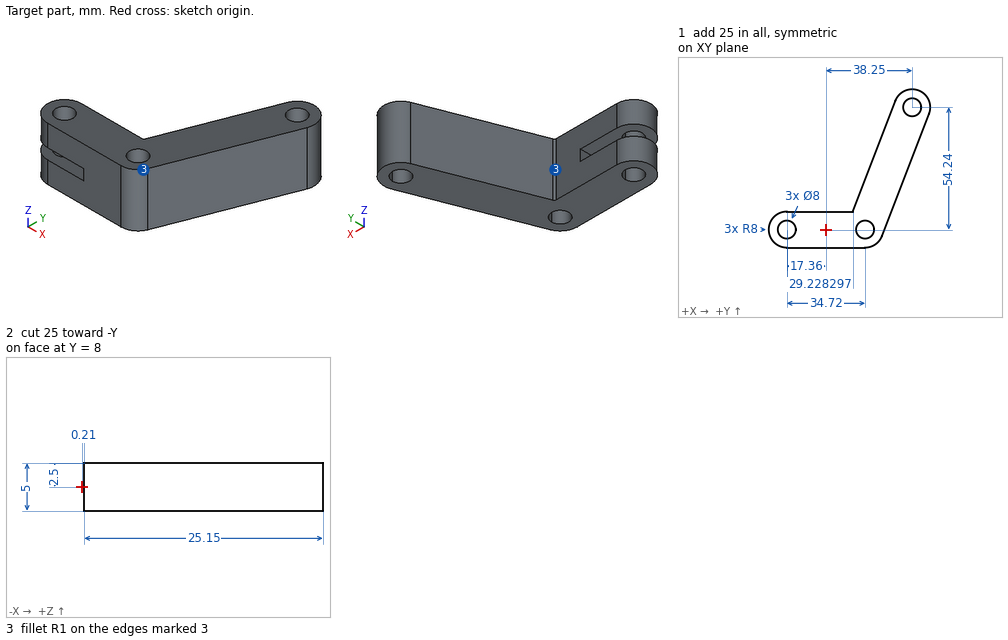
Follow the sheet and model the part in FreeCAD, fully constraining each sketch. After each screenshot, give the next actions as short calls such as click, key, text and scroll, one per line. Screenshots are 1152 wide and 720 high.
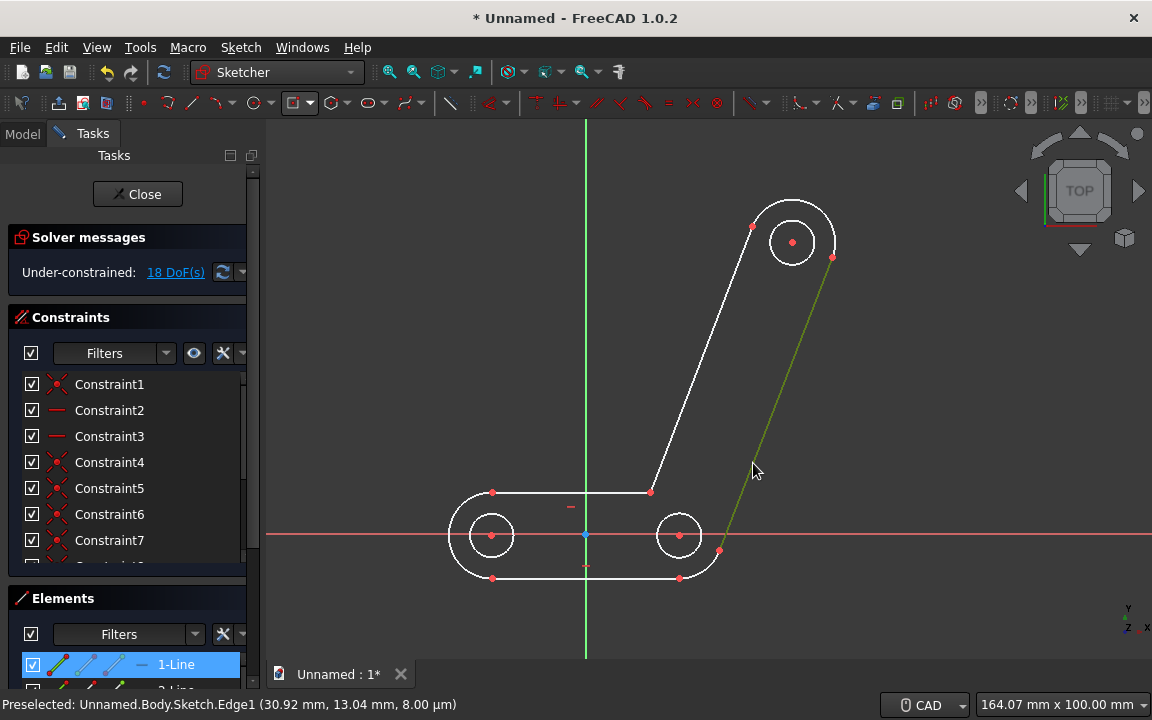
click(828, 219)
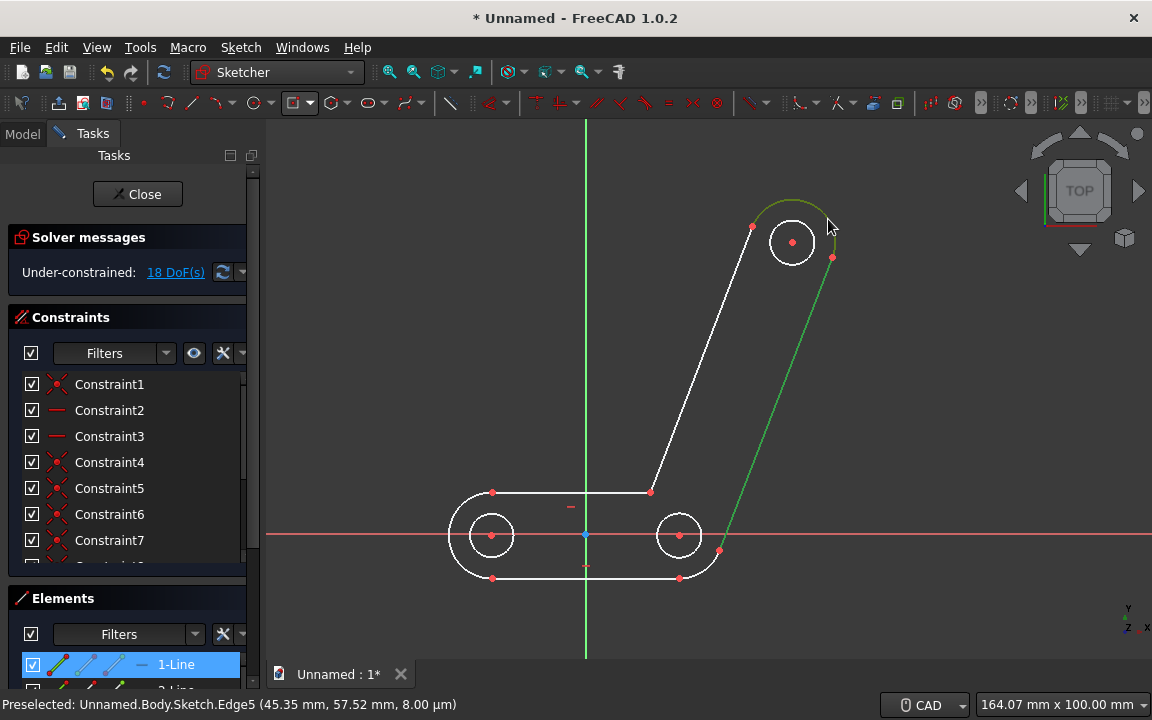
click(646, 104)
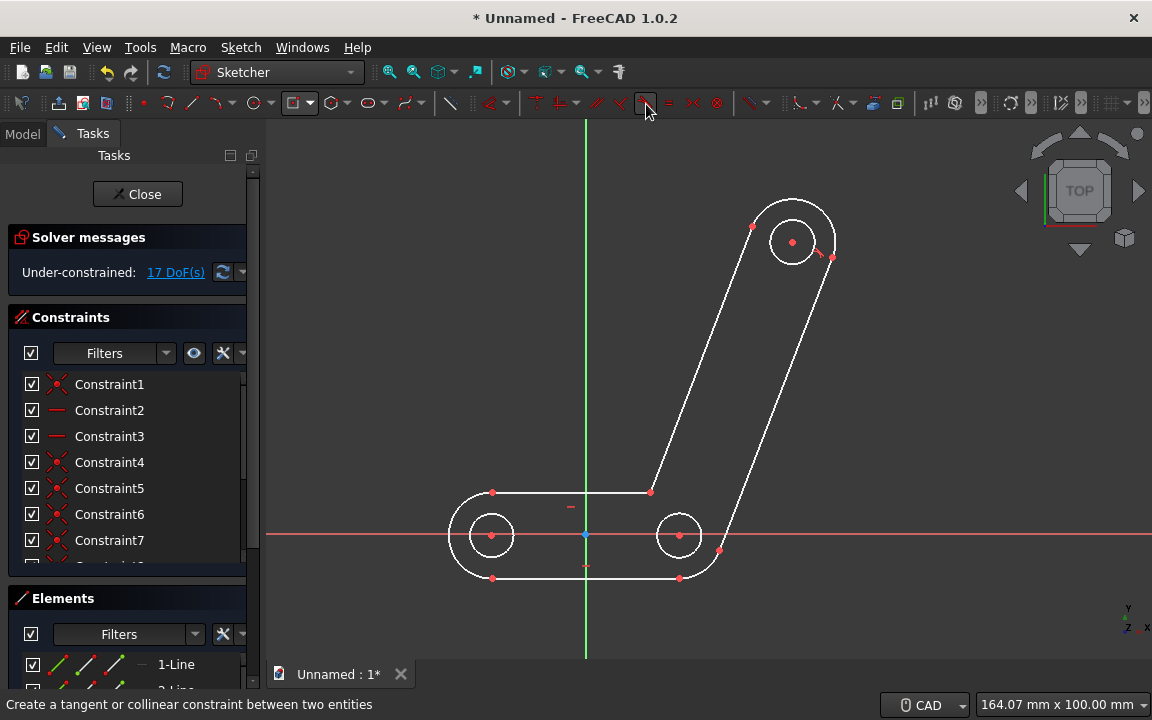
click(753, 463)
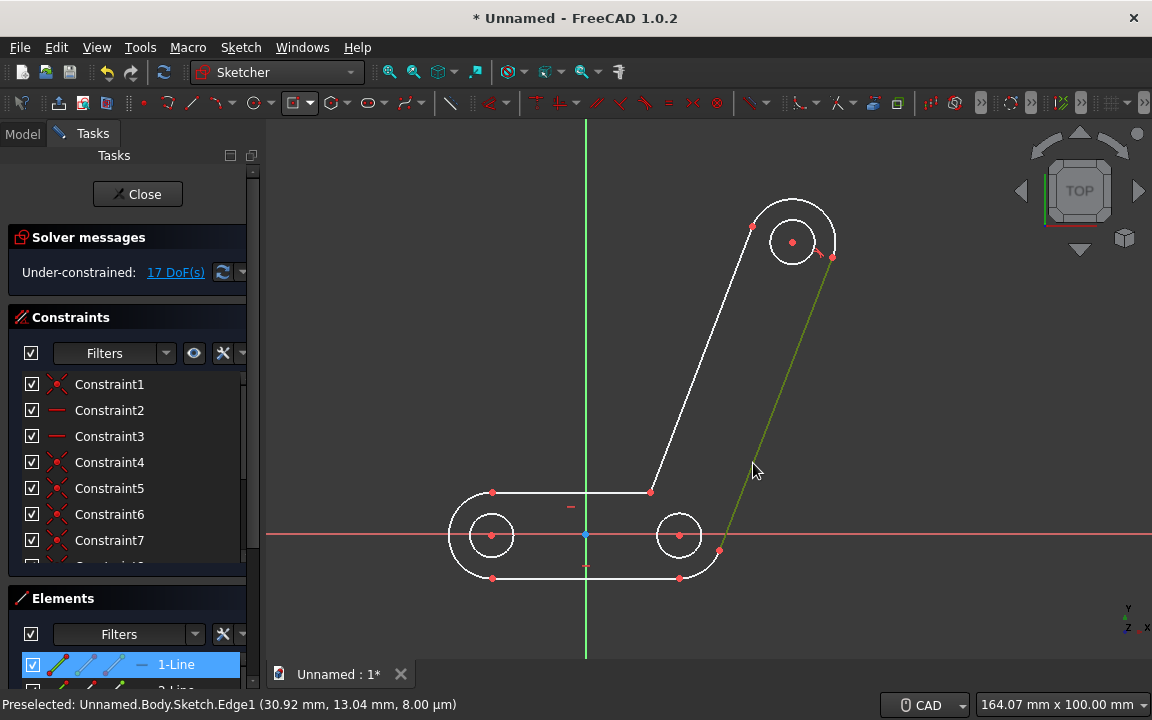
click(695, 576)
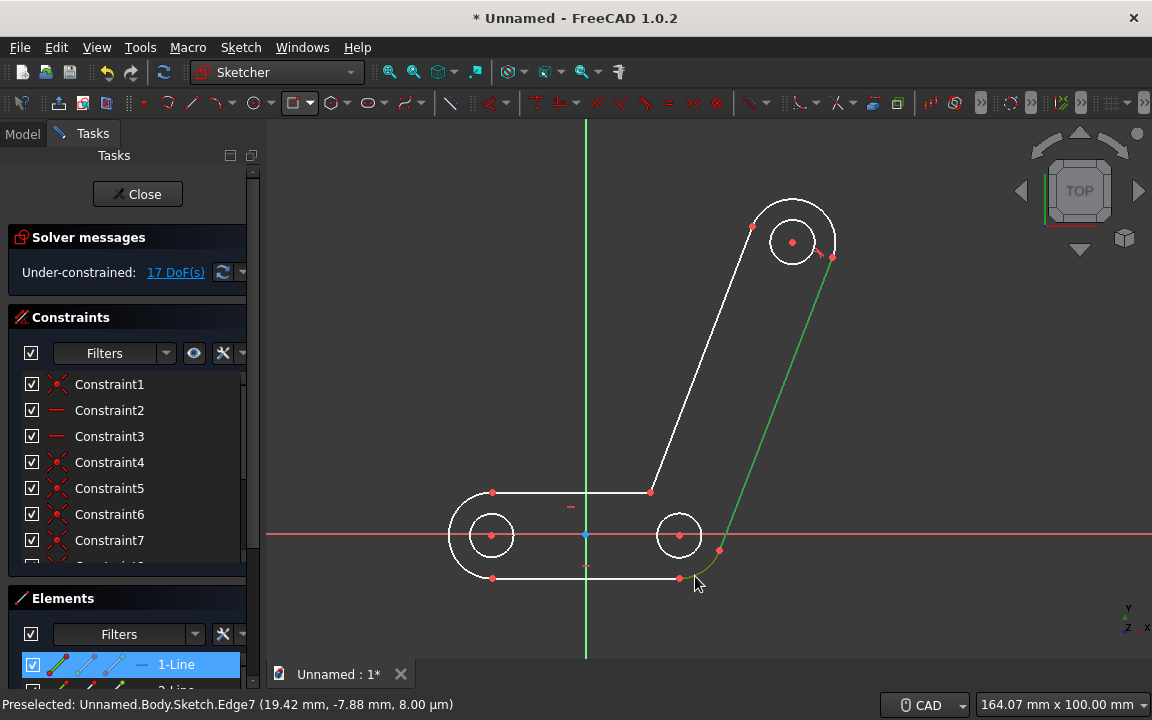
click(646, 104)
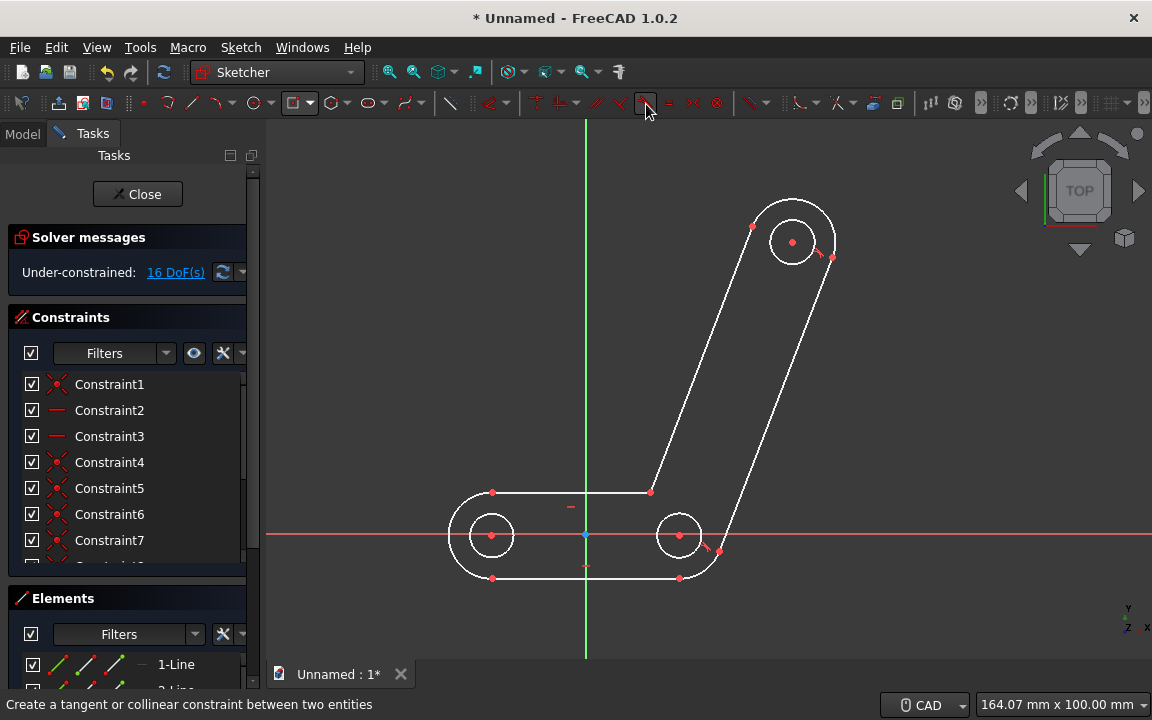
click(722, 306)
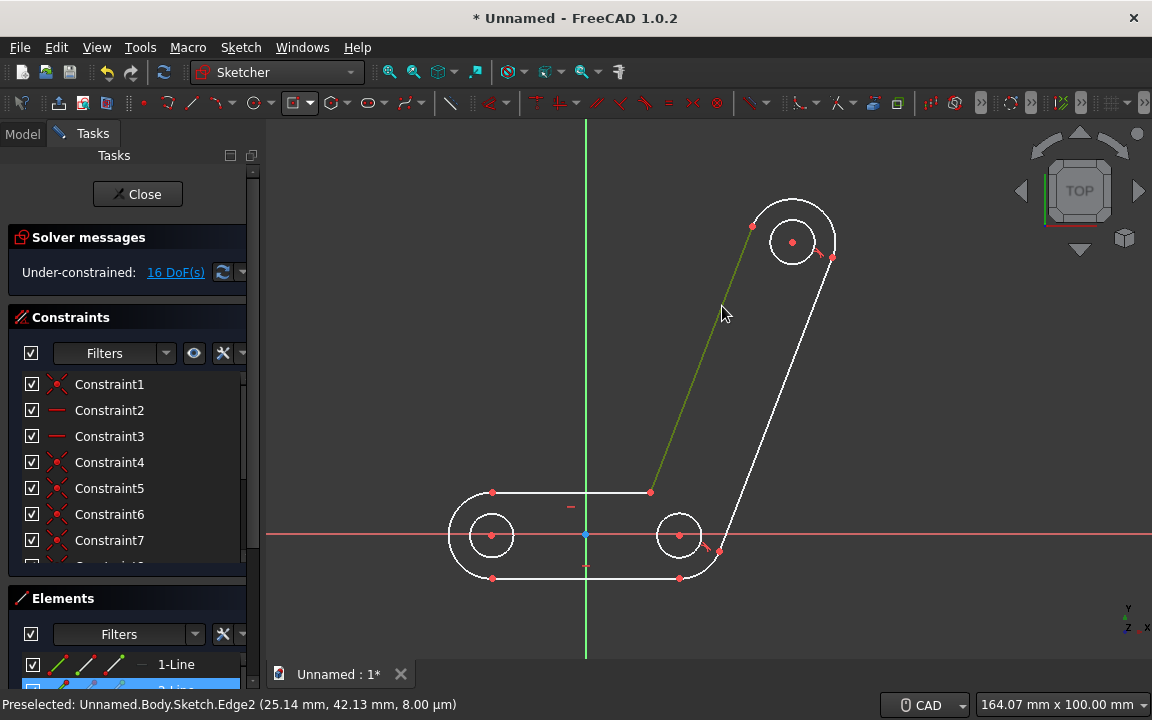
click(829, 219)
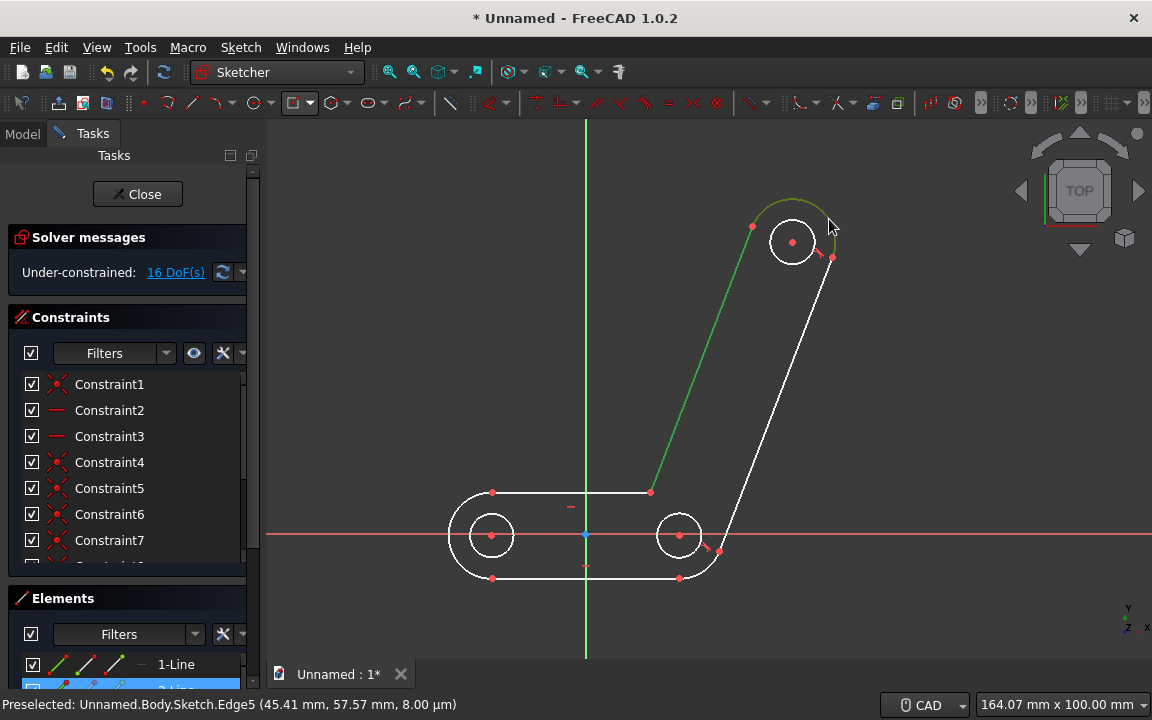
click(646, 104)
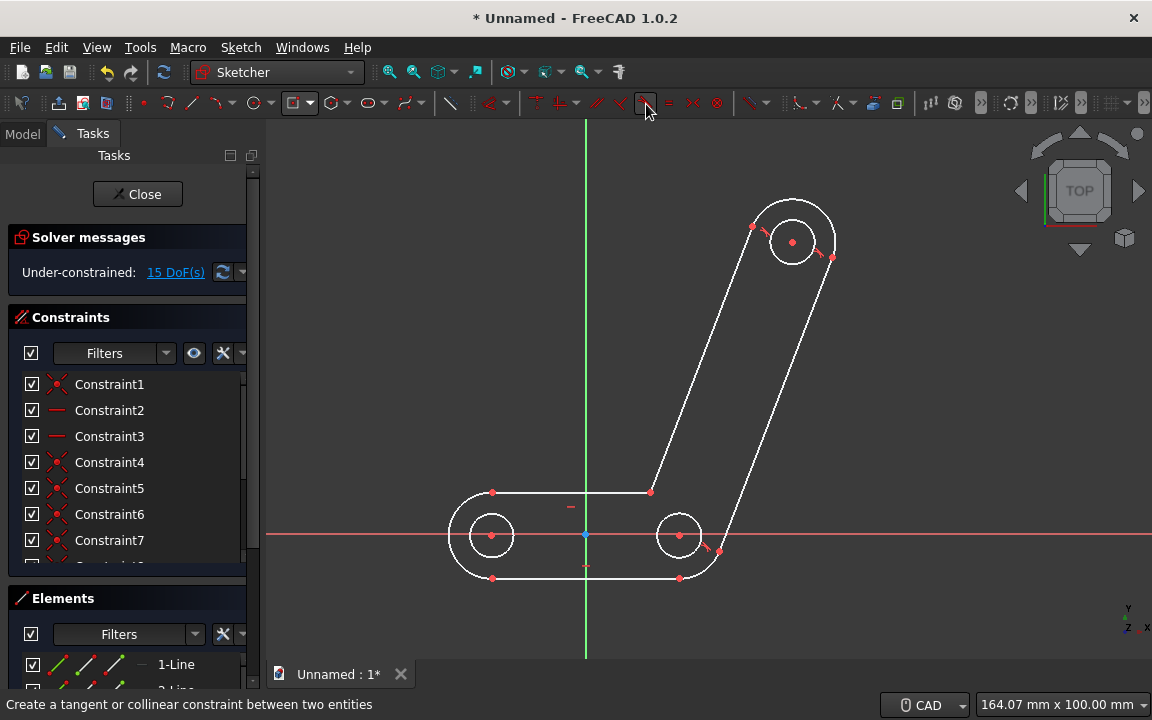
click(603, 493)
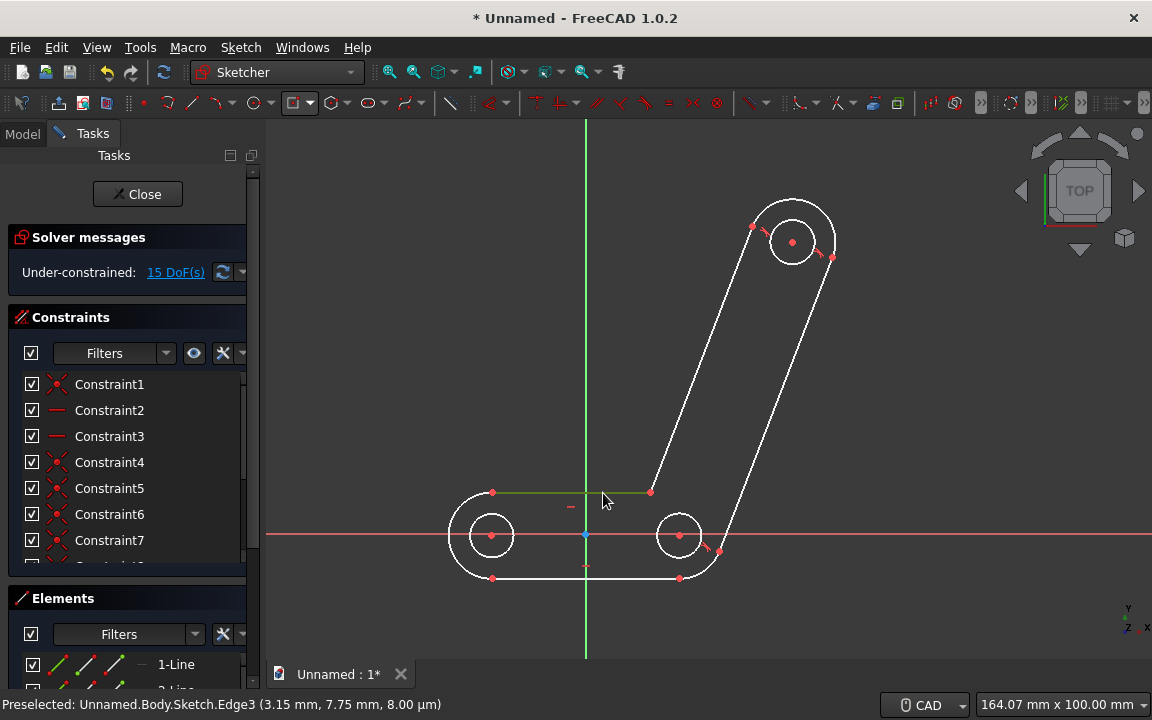
click(457, 510)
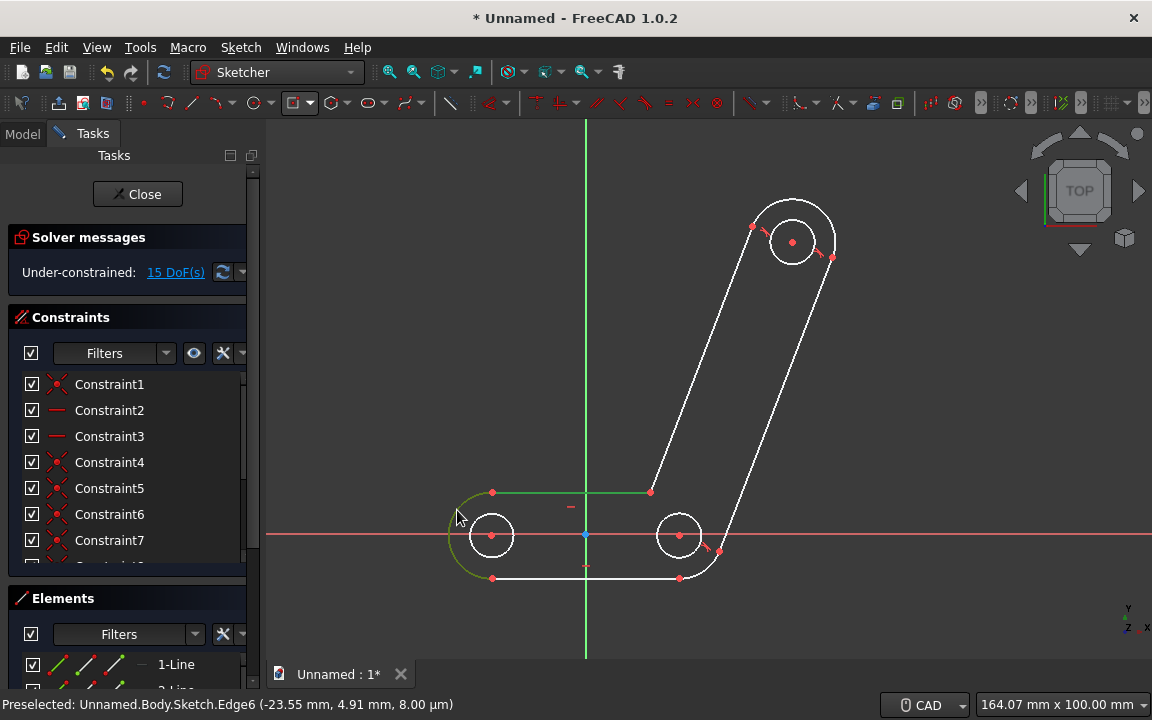
click(646, 104)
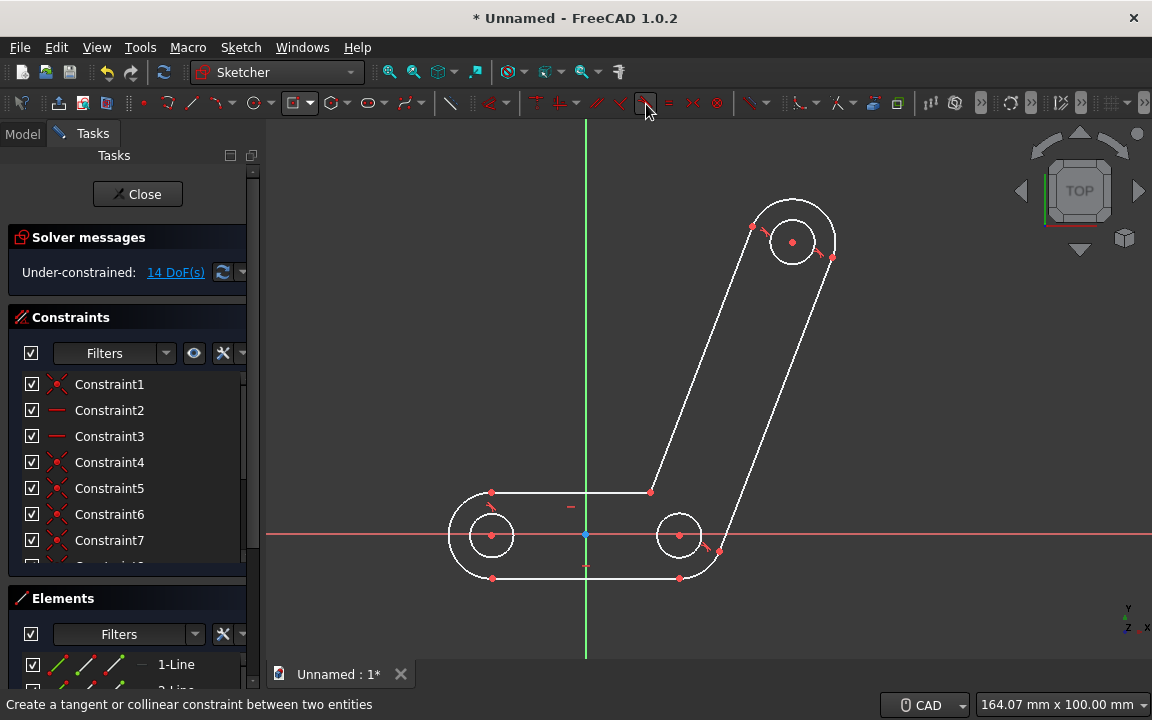
click(549, 579)